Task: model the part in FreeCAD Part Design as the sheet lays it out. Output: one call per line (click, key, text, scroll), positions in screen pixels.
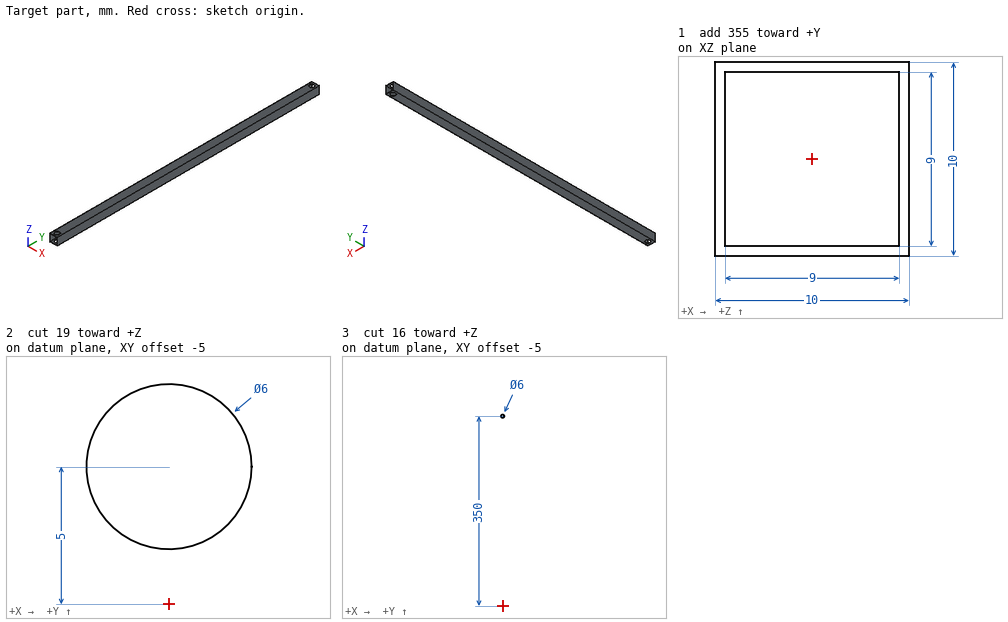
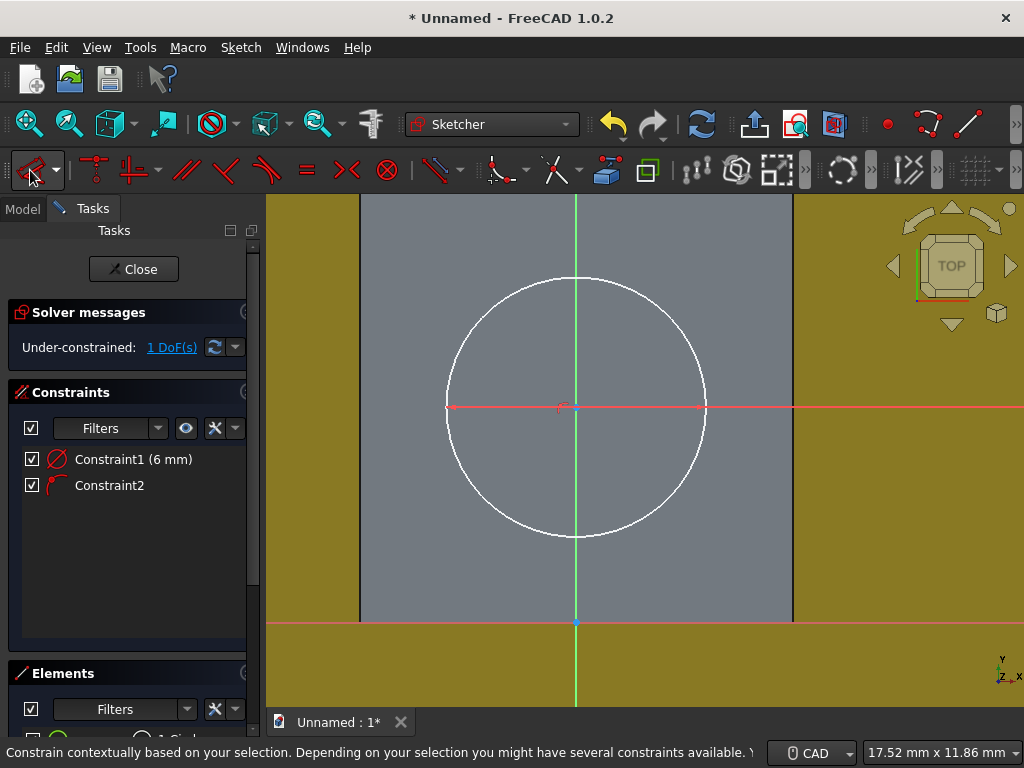
click(576, 407)
click(610, 515)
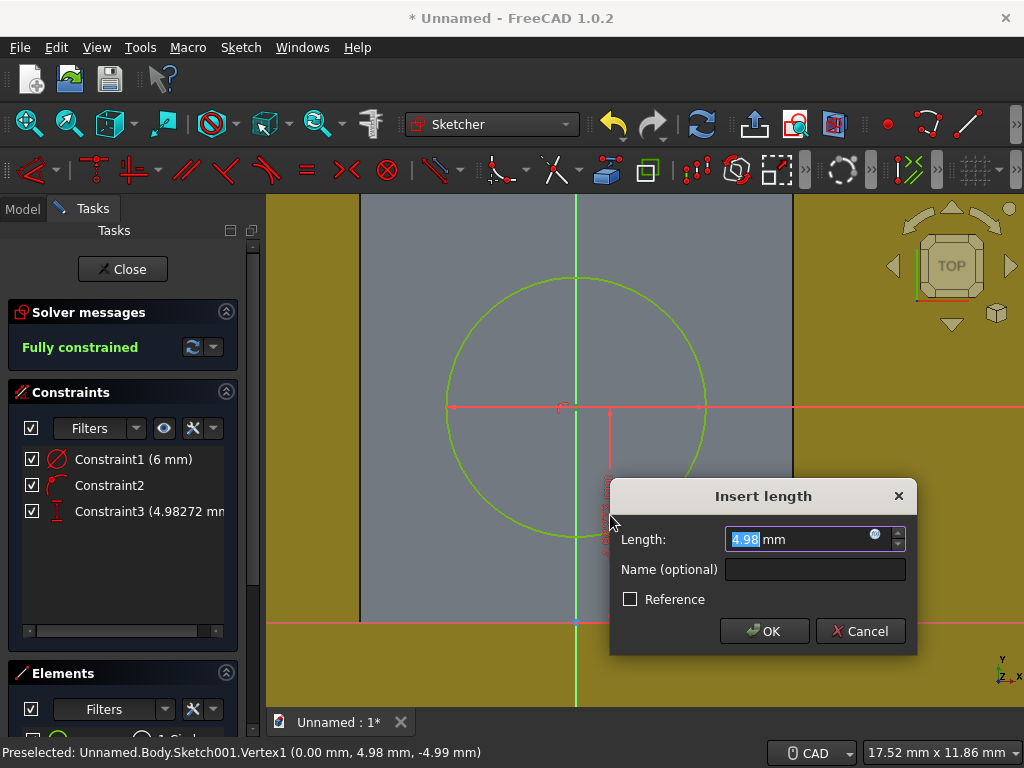
text(5)
key(Return)
key(Escape)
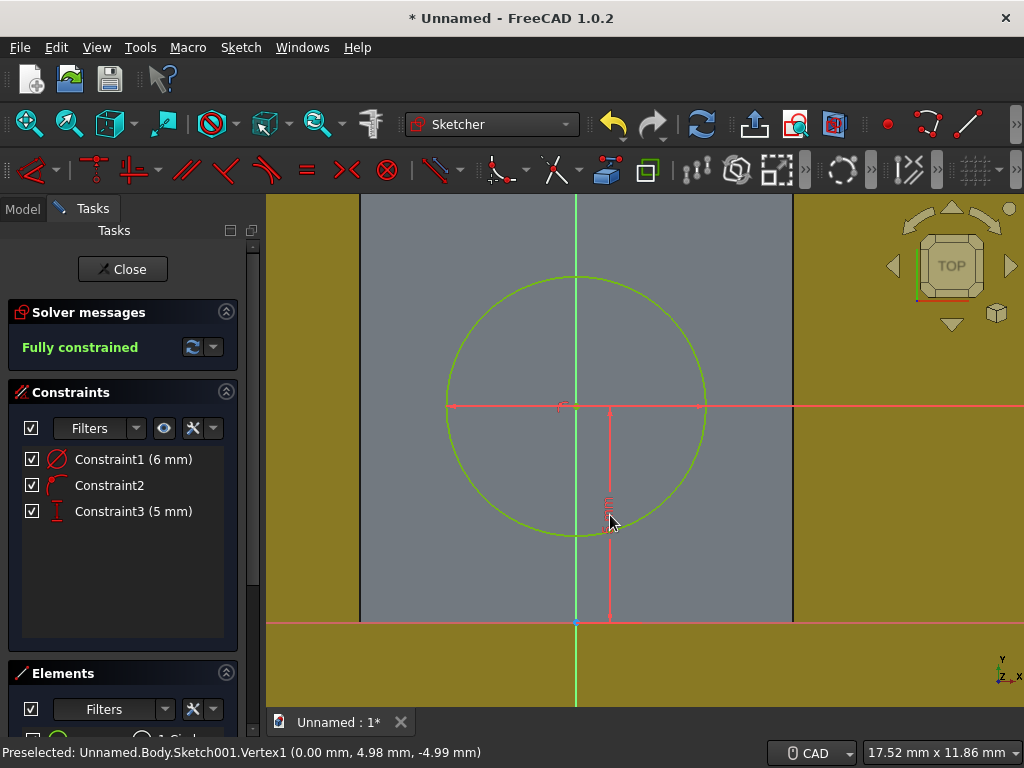
click(123, 269)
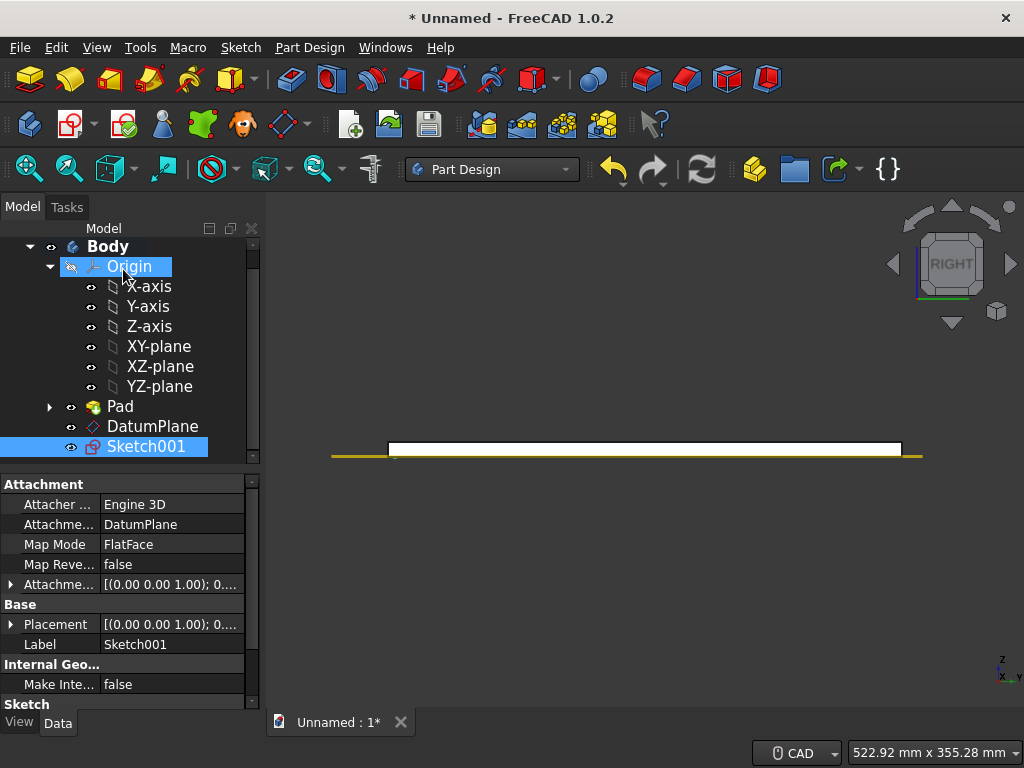
click(292, 80)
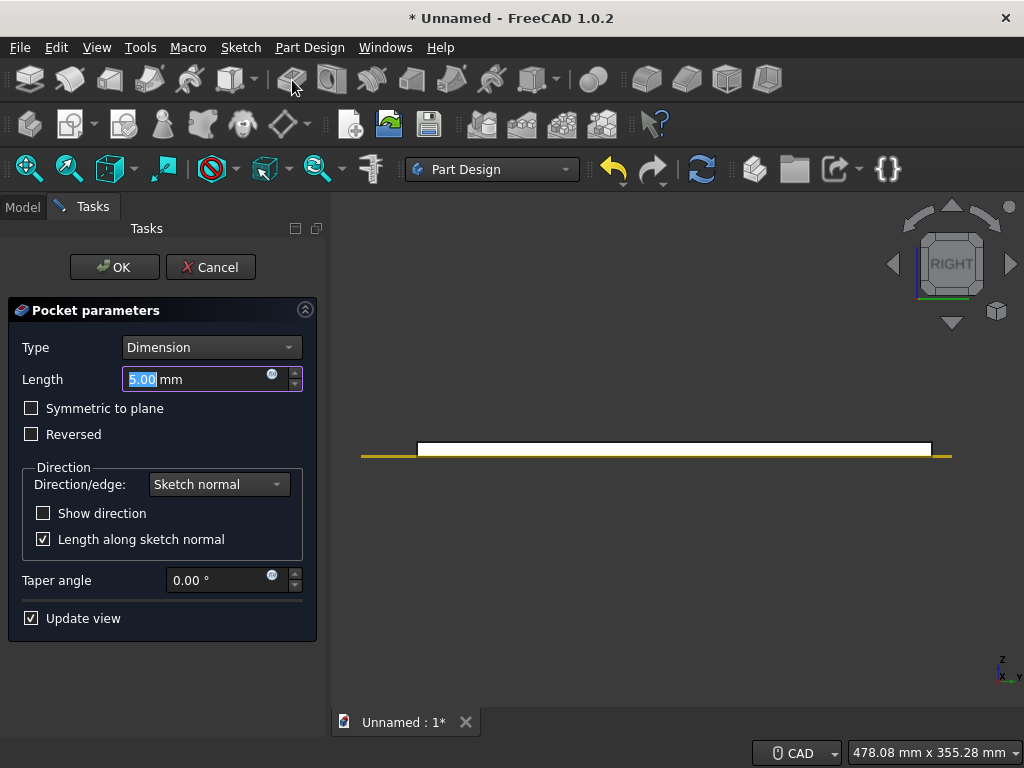
text(19)
key(Tab)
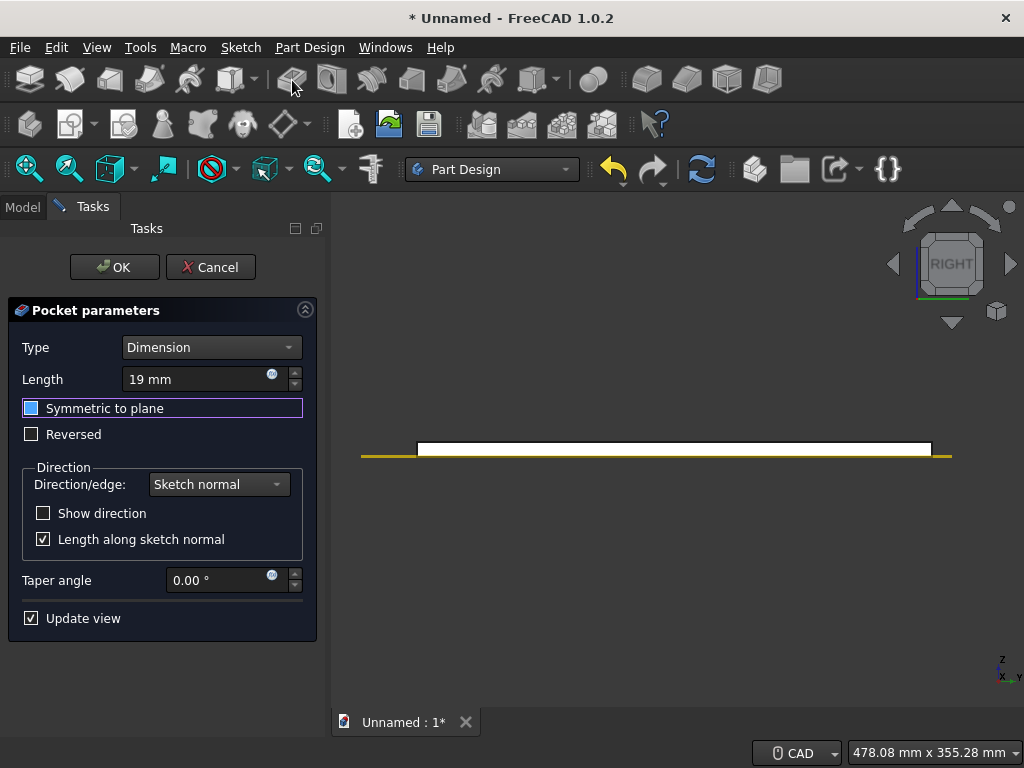
click(30, 434)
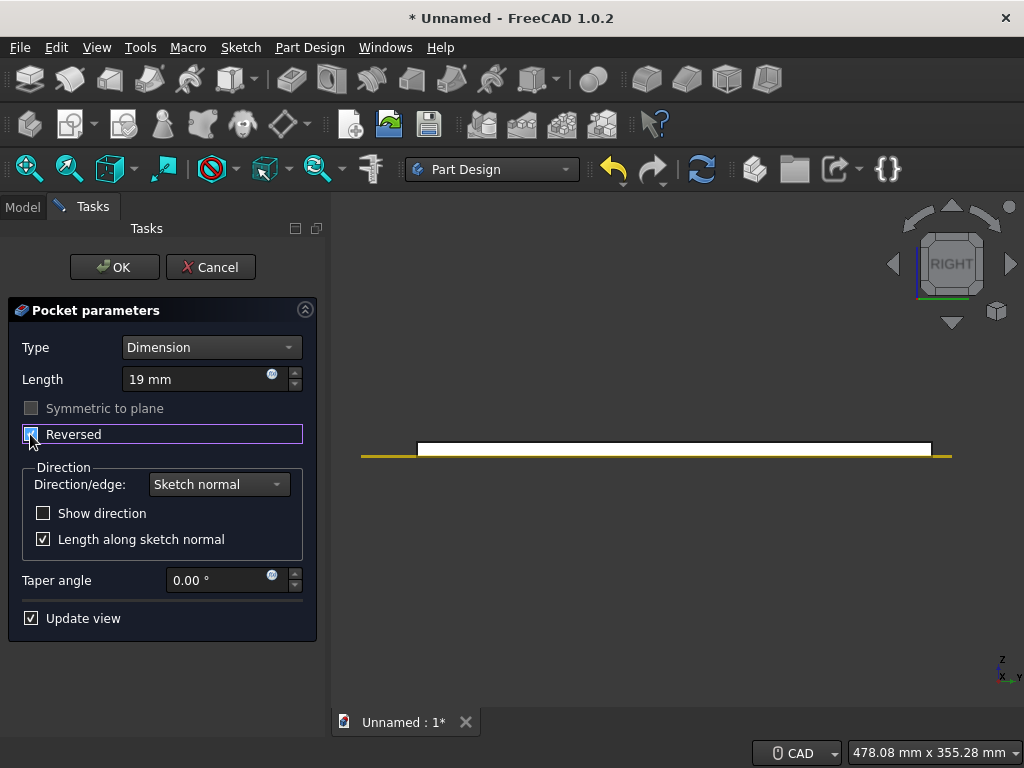
click(115, 267)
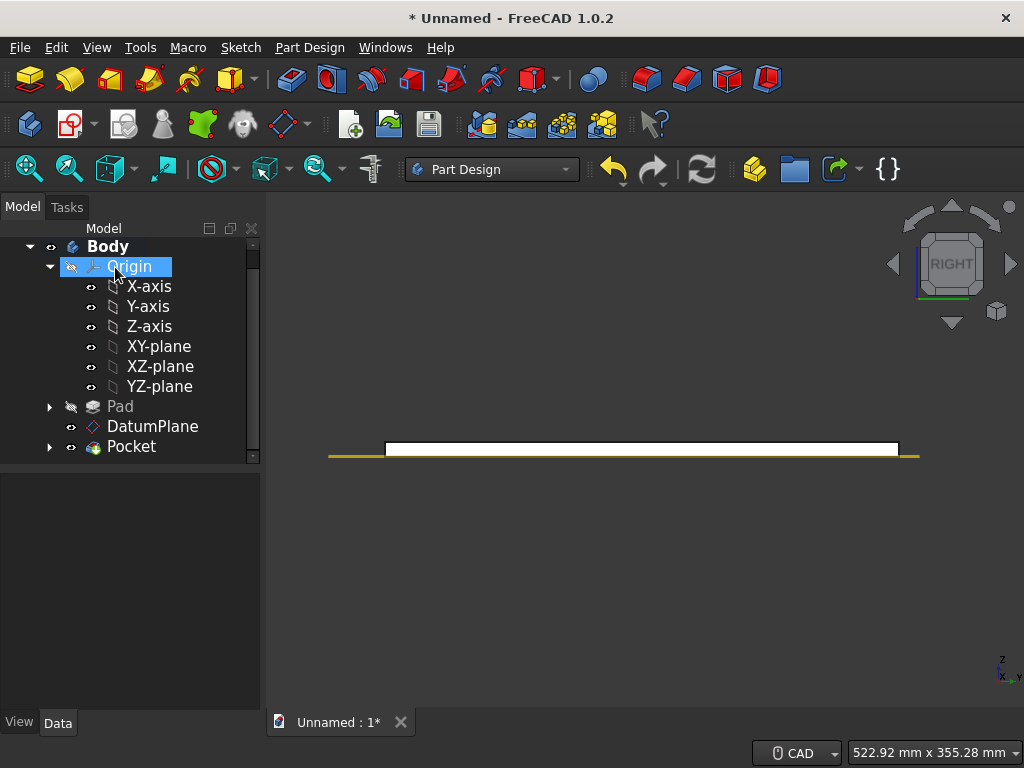
click(116, 427)
key(space)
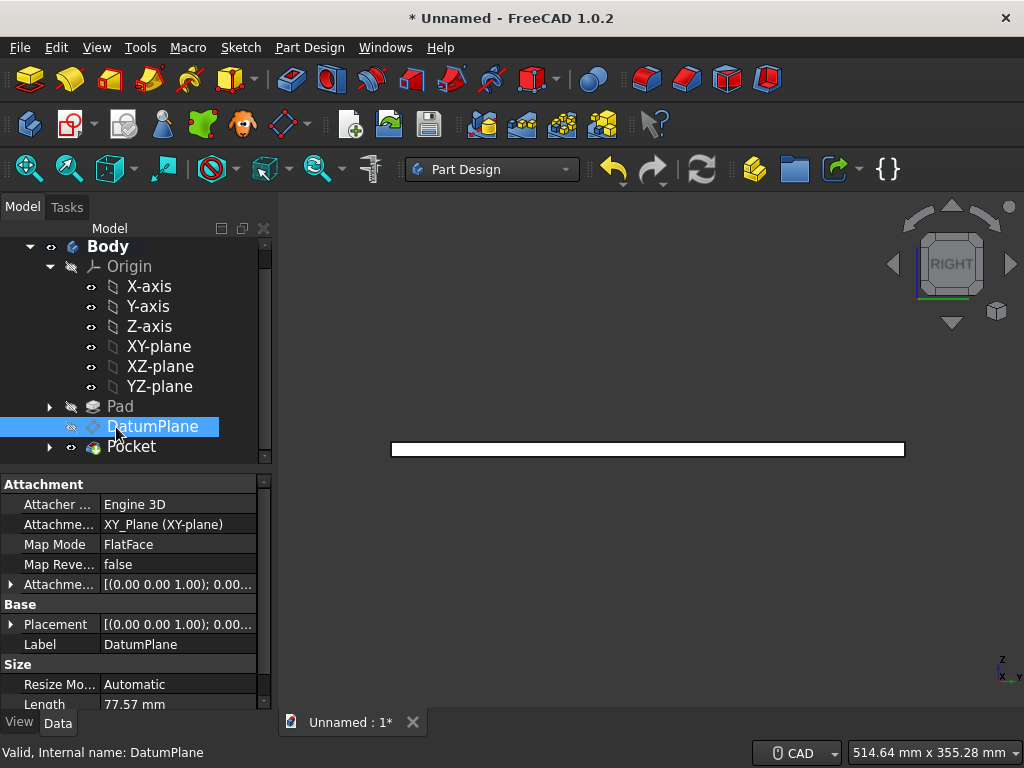
key(5)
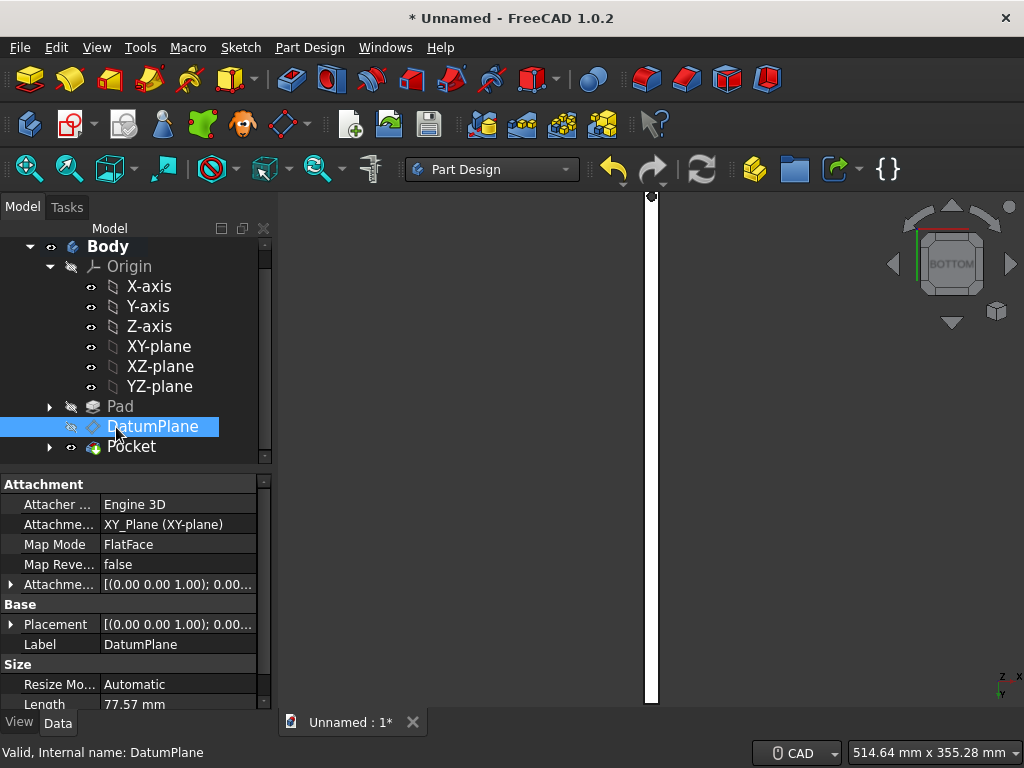
click(30, 170)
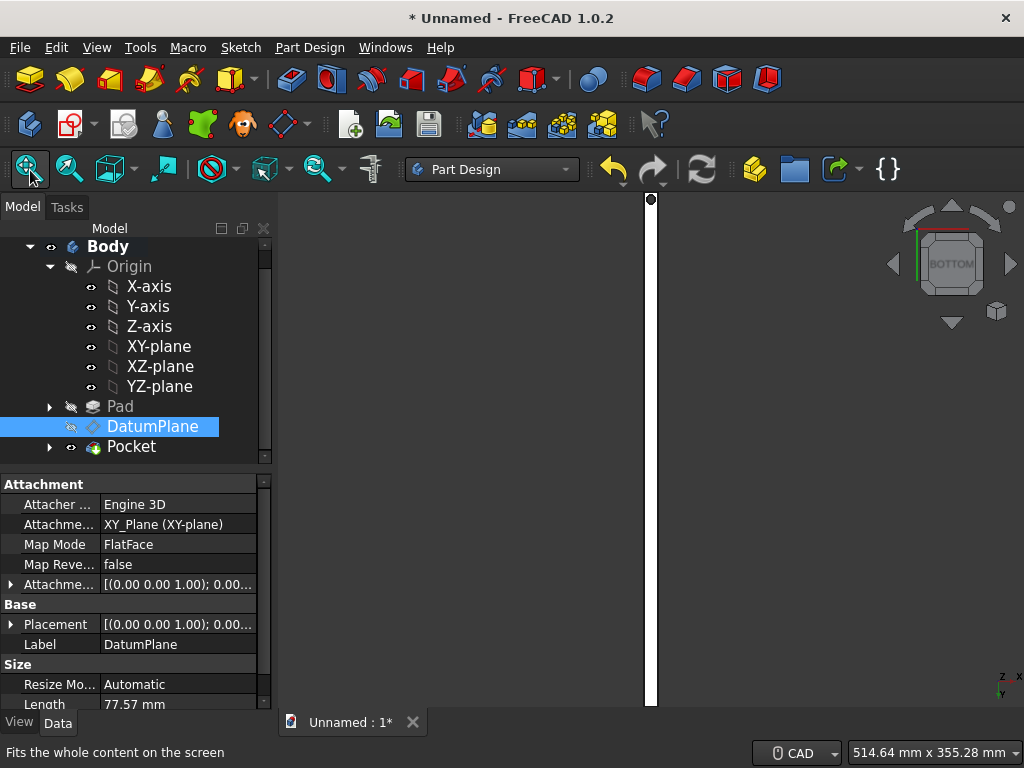
key(1)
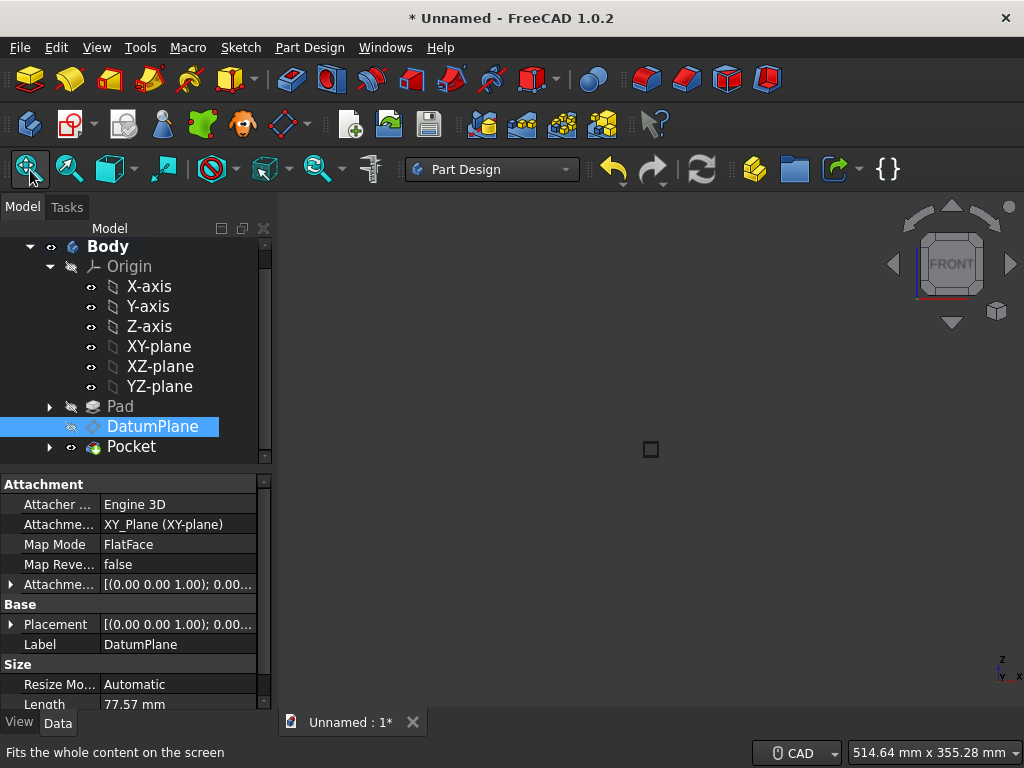
click(30, 170)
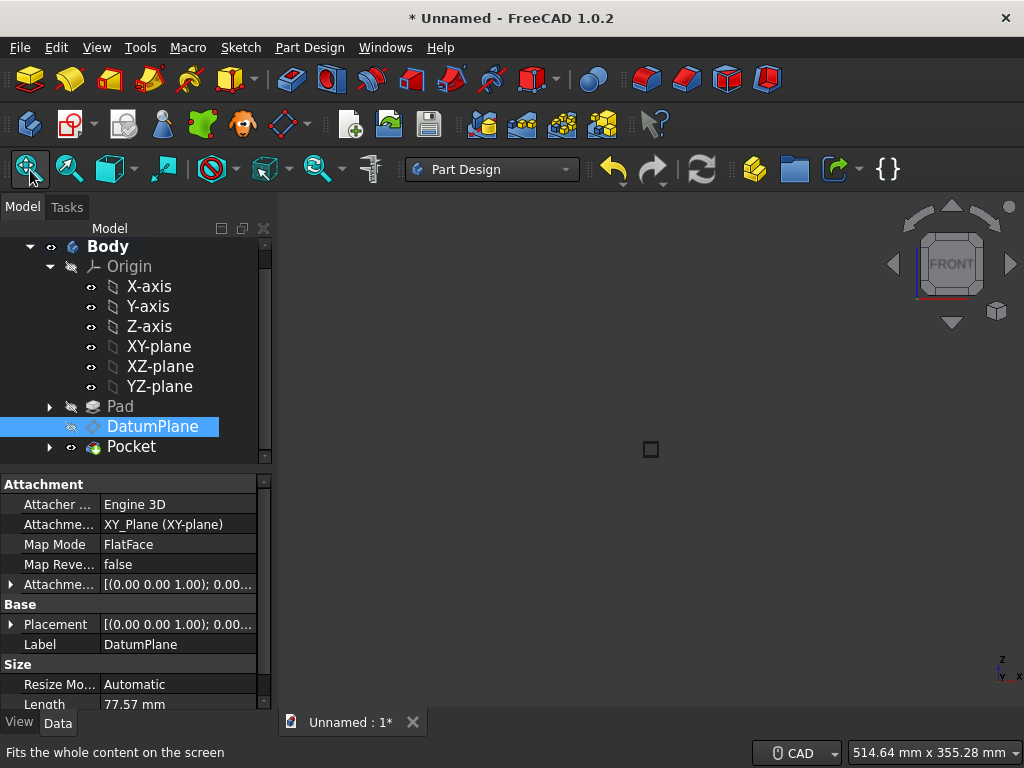
key(3)